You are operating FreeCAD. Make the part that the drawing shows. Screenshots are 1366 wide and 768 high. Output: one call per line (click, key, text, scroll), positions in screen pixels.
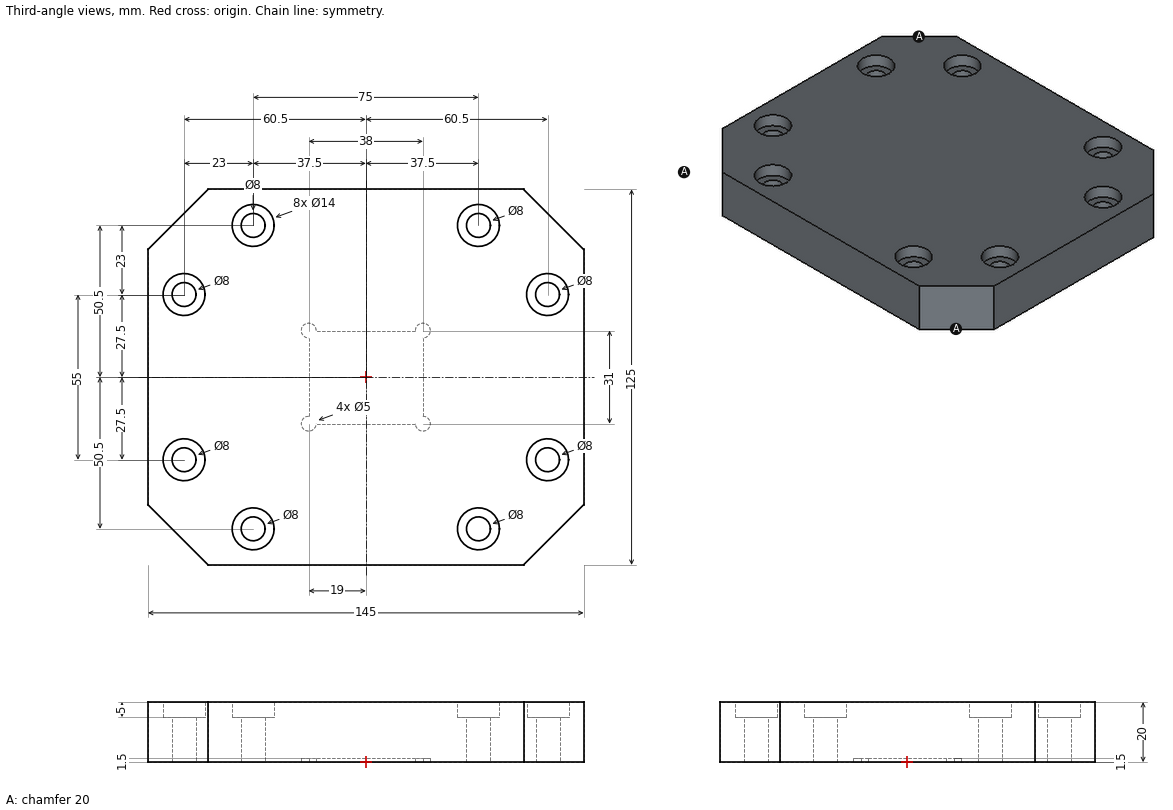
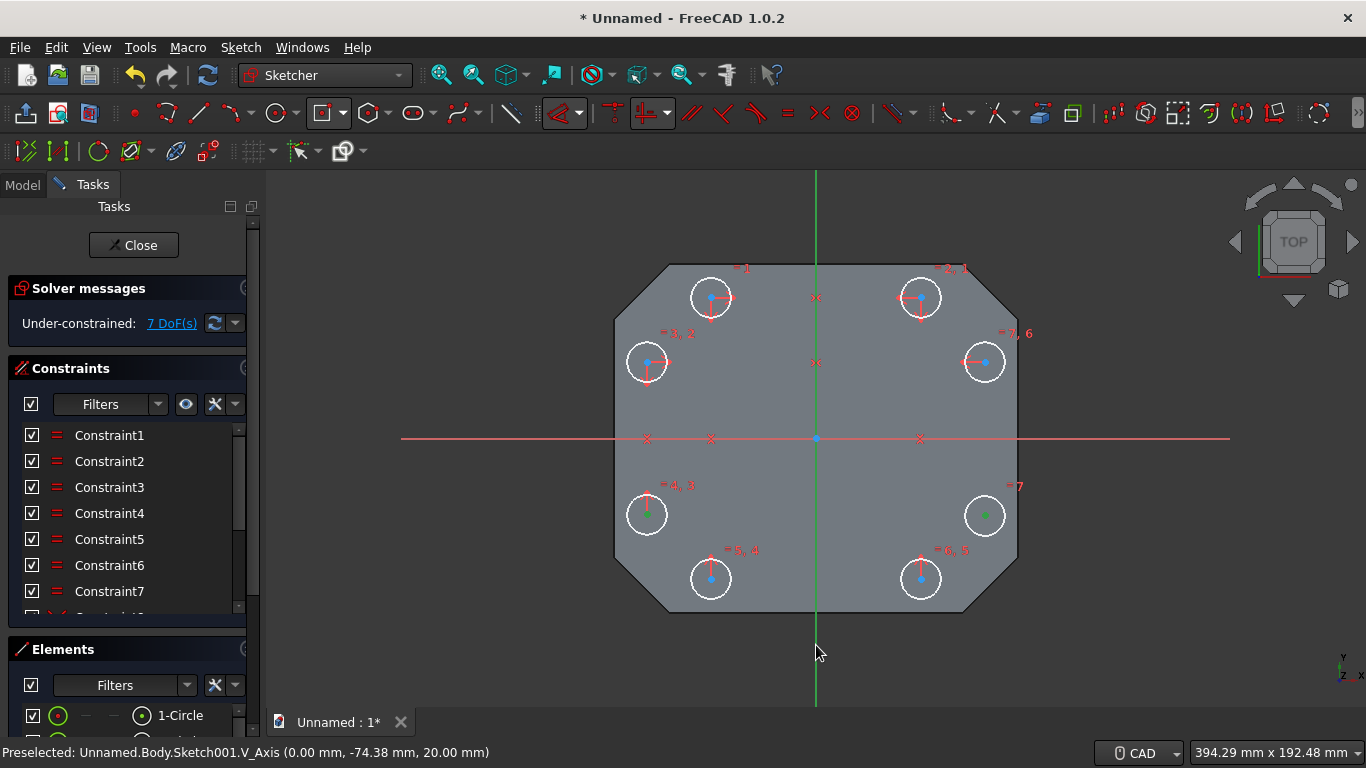
key(s)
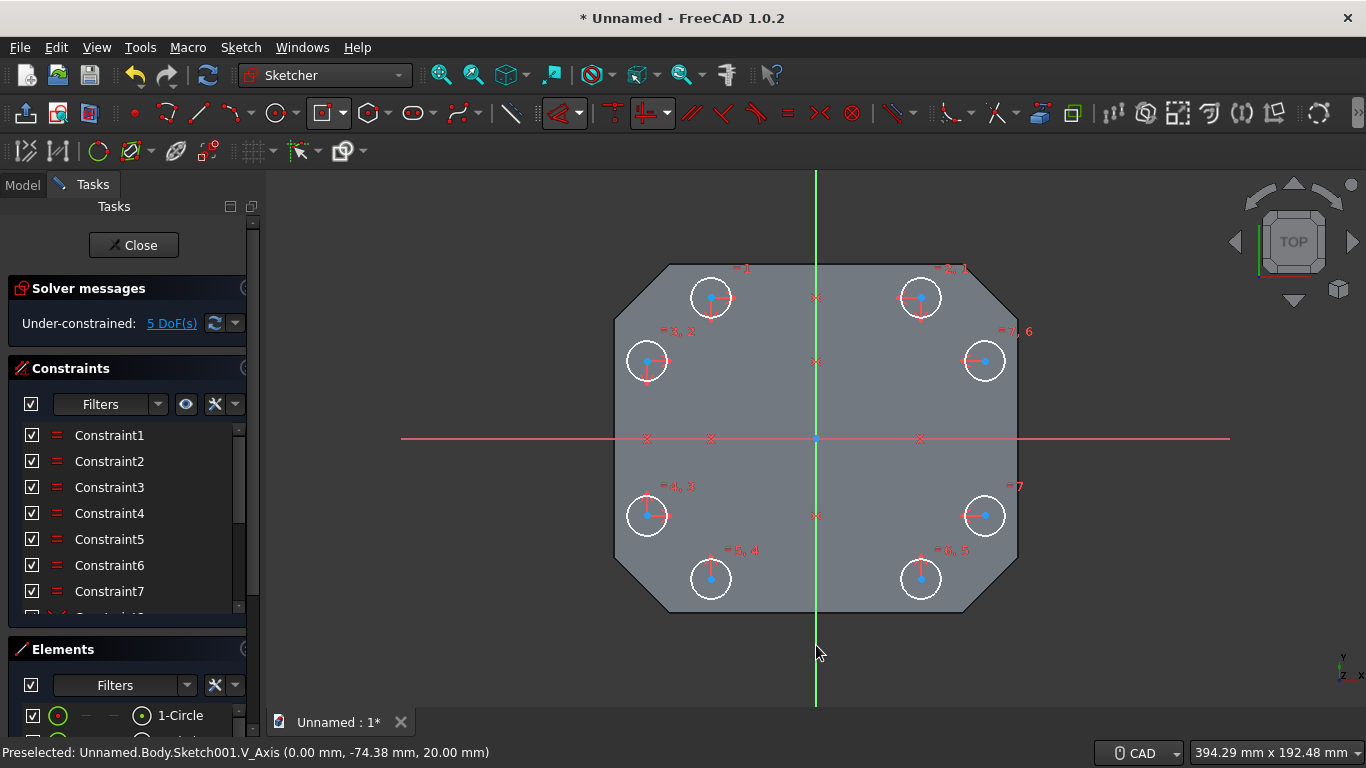
click(725, 284)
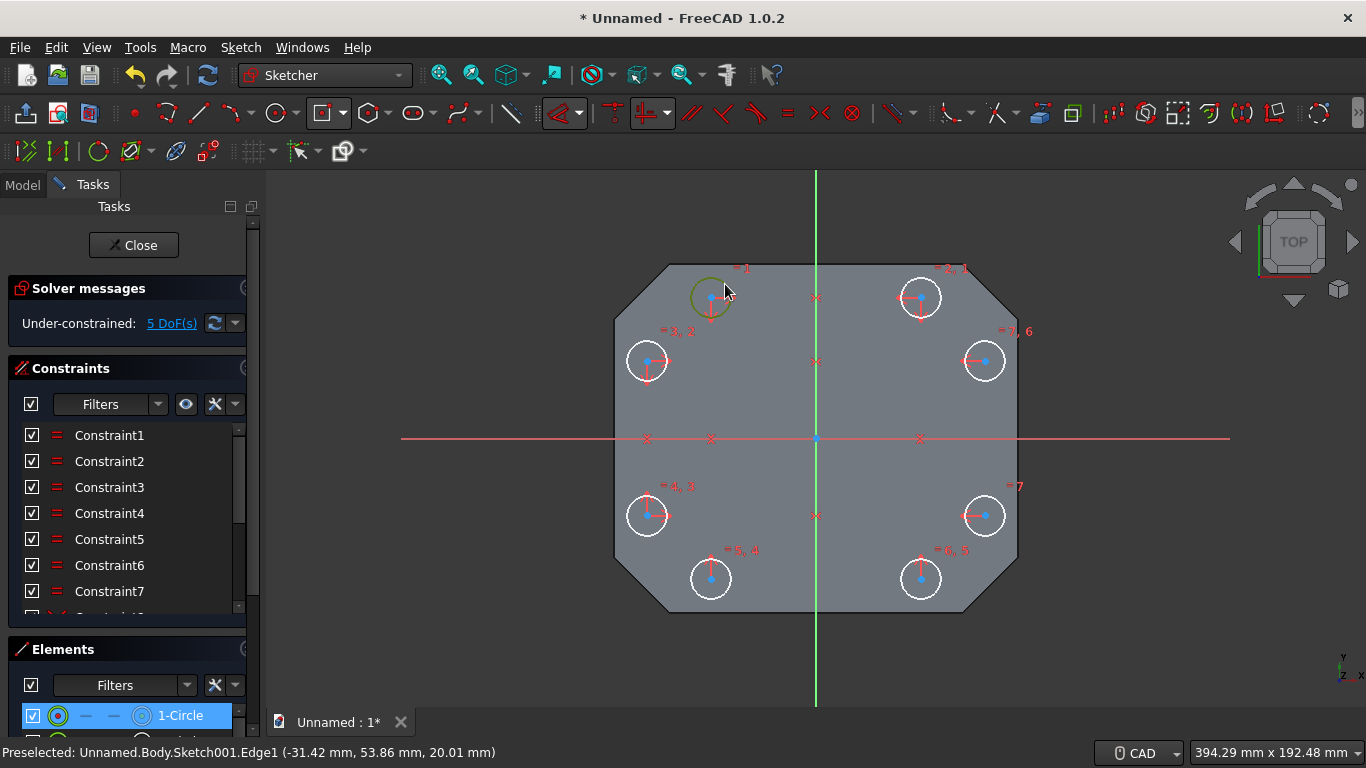
key(k)
key(o)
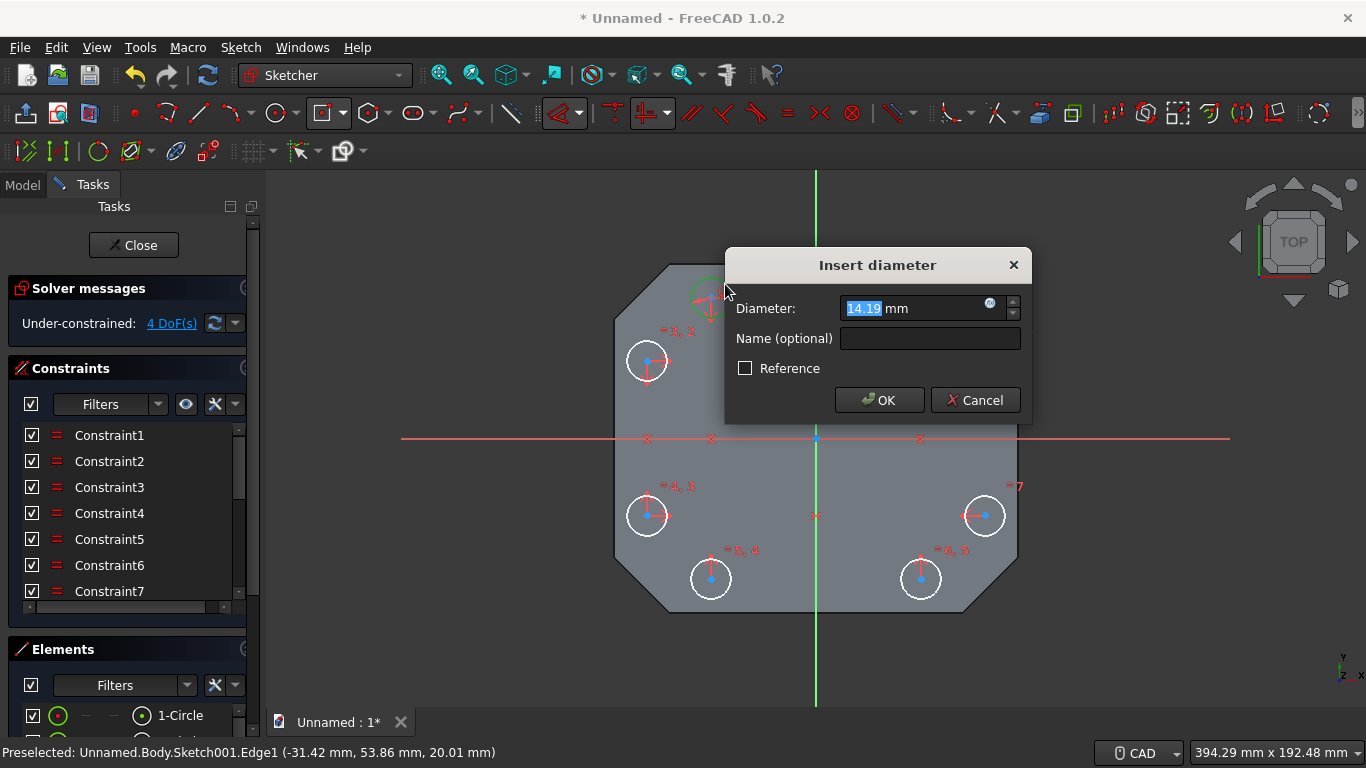
text(14)
key(Return)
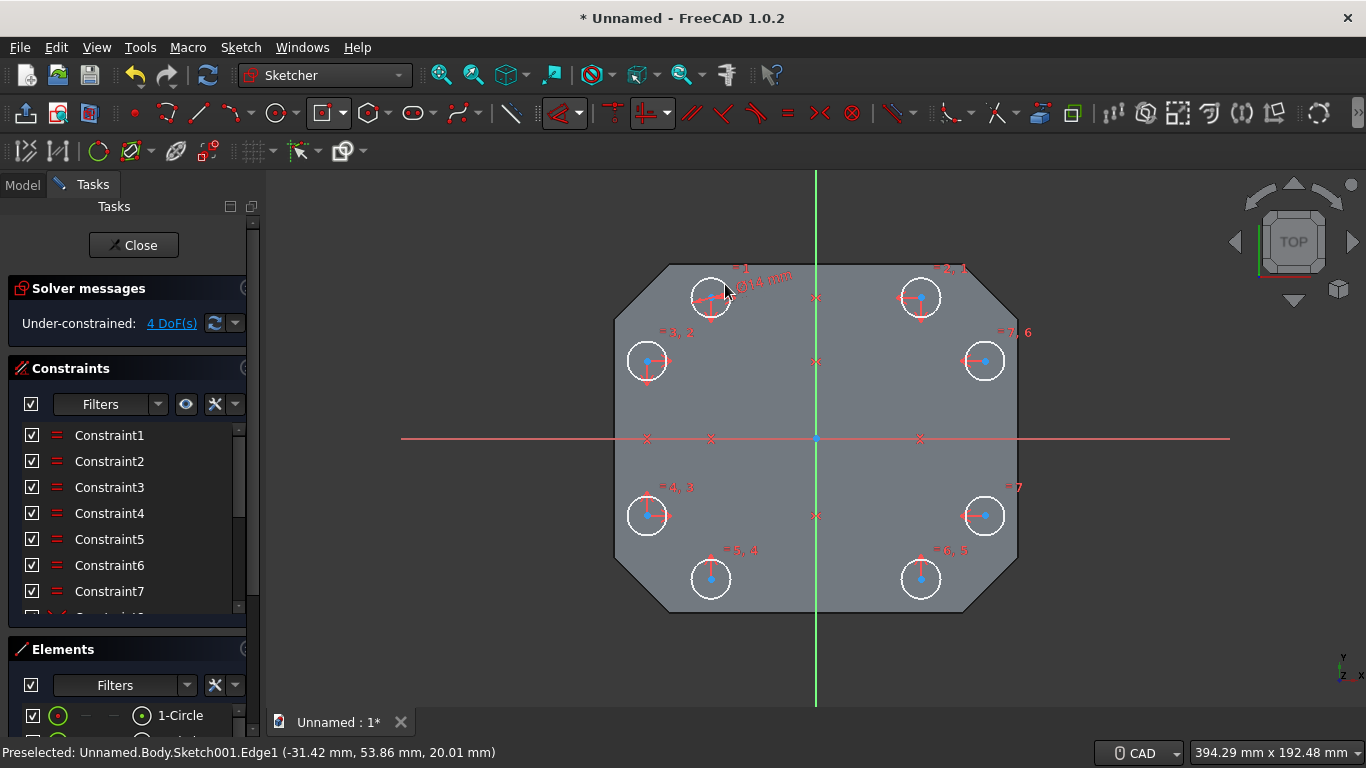
click(711, 298)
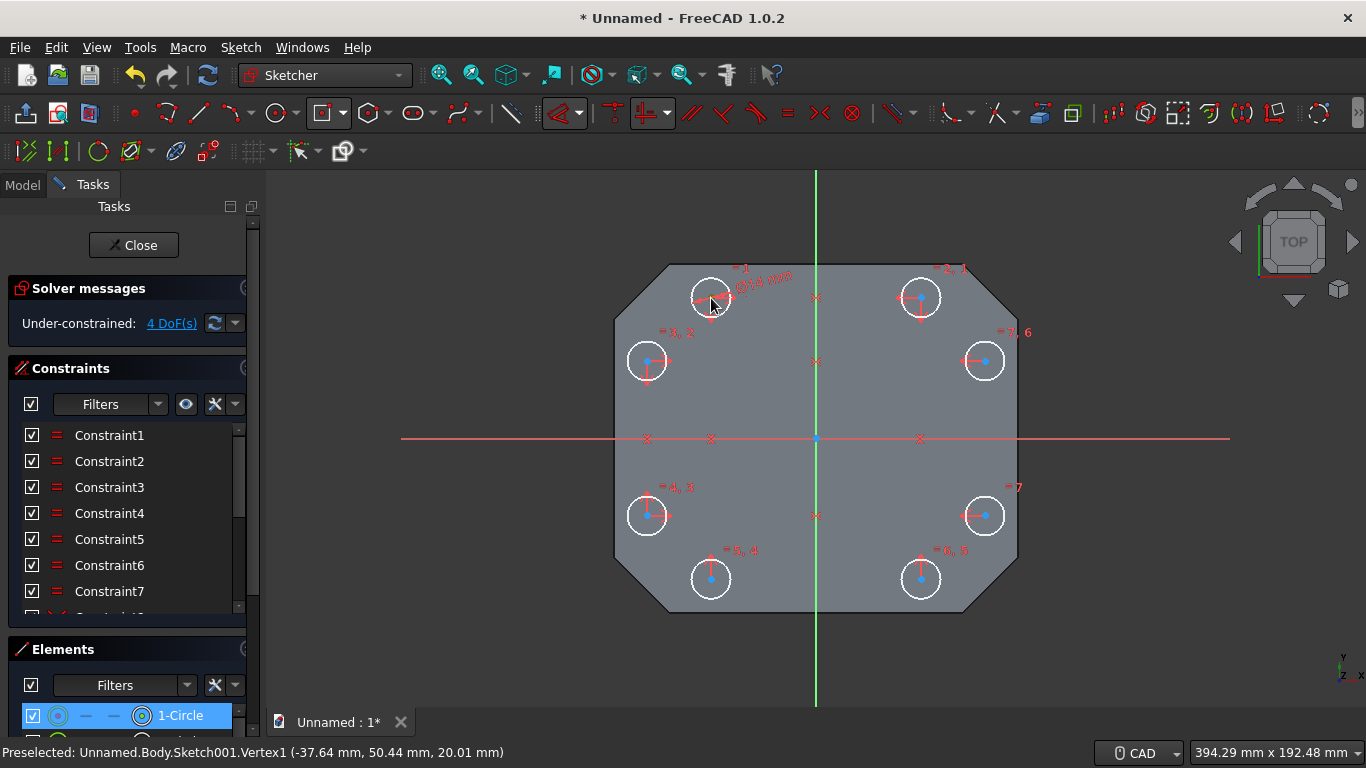
click(921, 298)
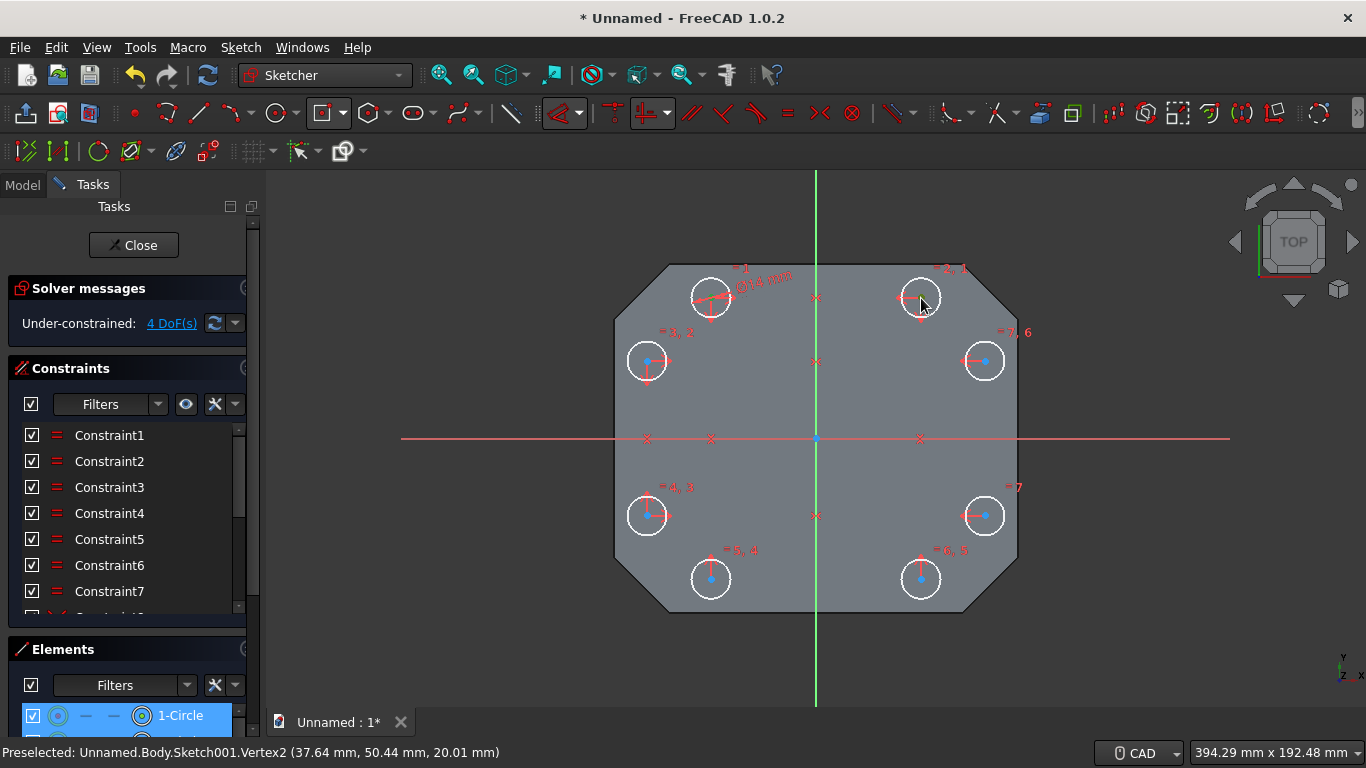
key(l)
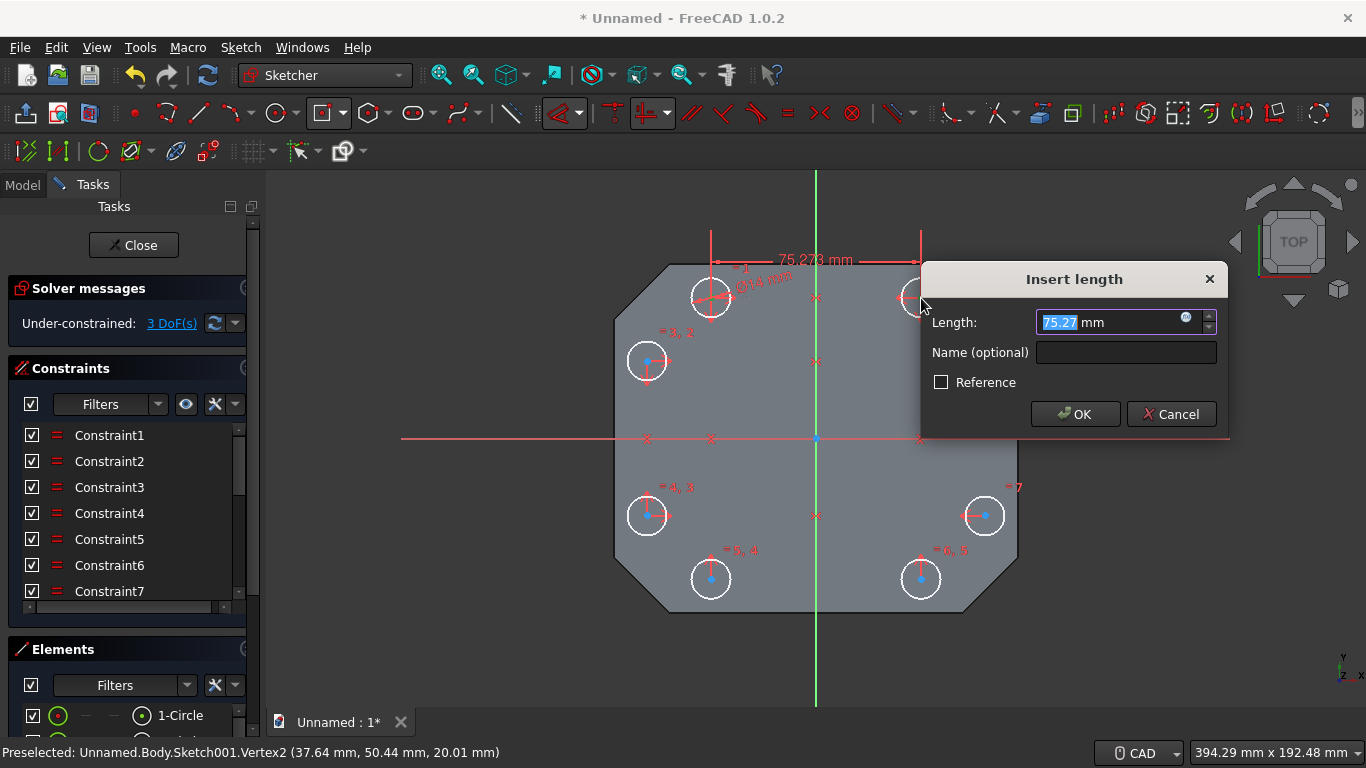
text(75)
key(Return)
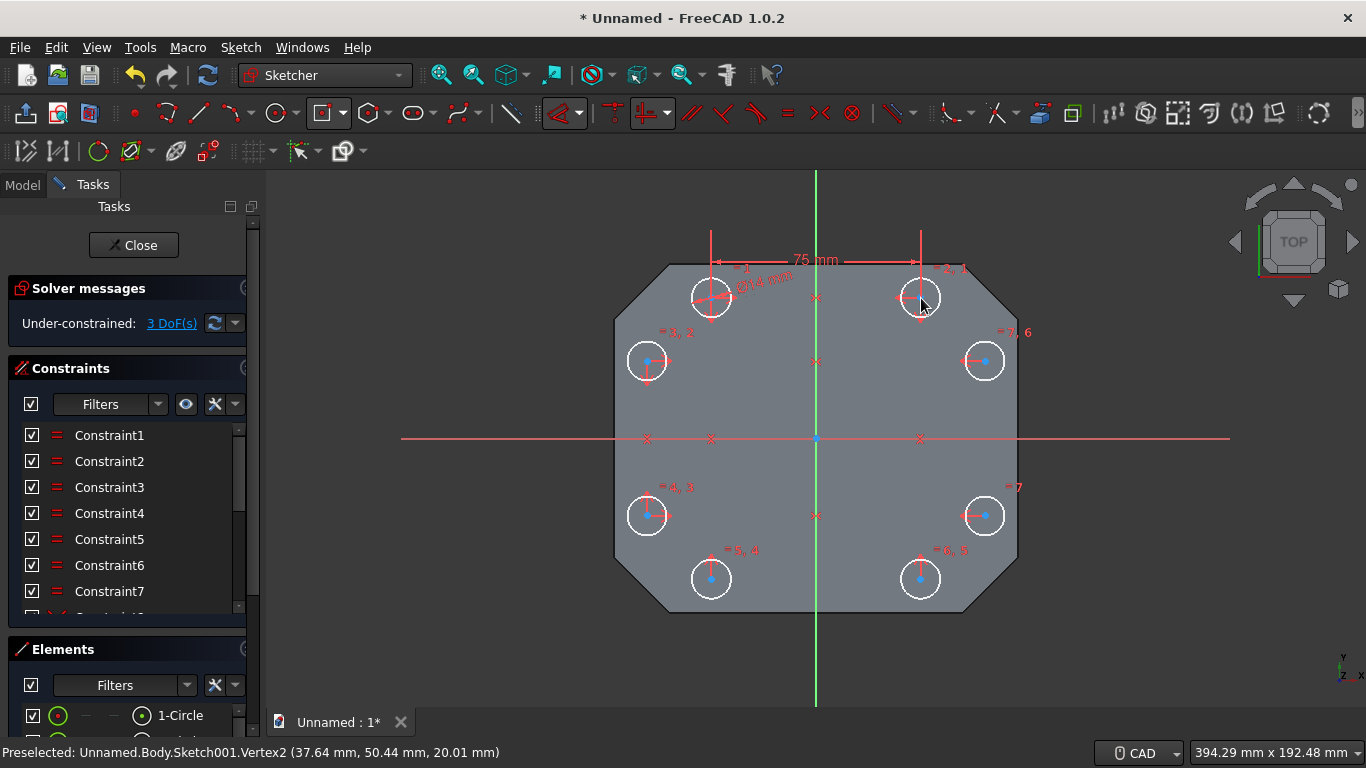
click(711, 298)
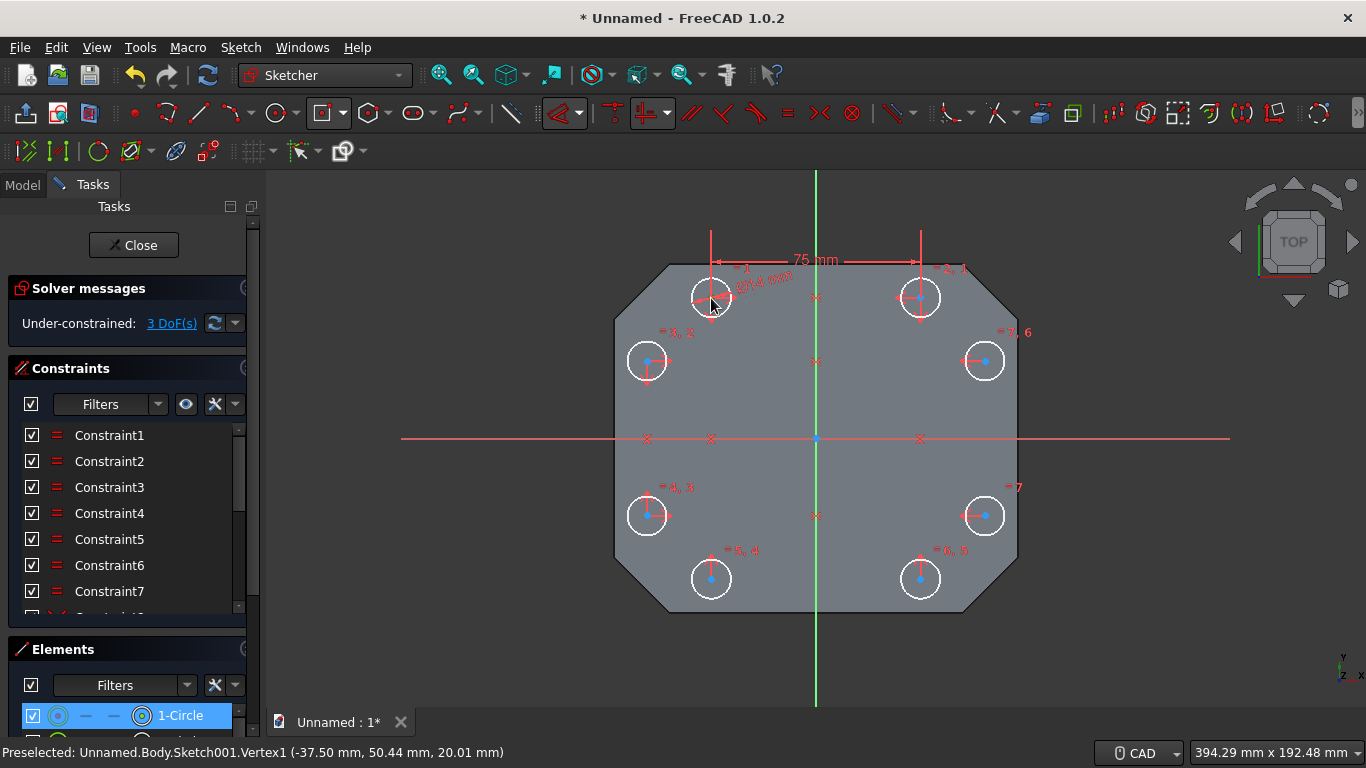
click(647, 361)